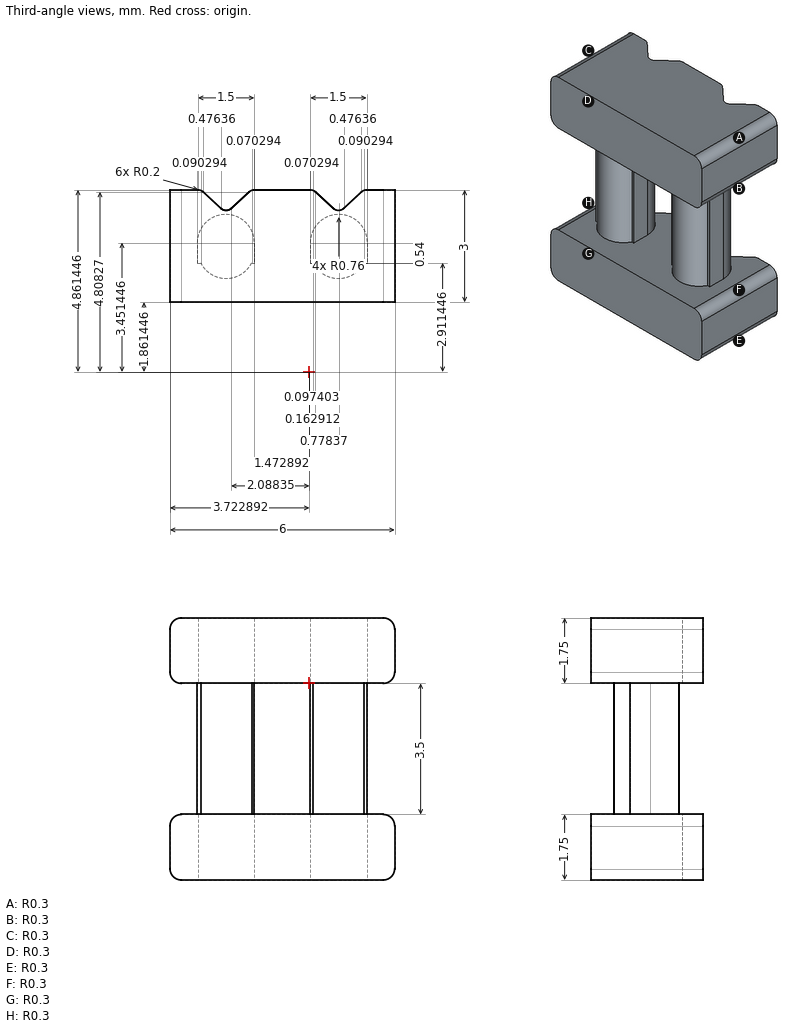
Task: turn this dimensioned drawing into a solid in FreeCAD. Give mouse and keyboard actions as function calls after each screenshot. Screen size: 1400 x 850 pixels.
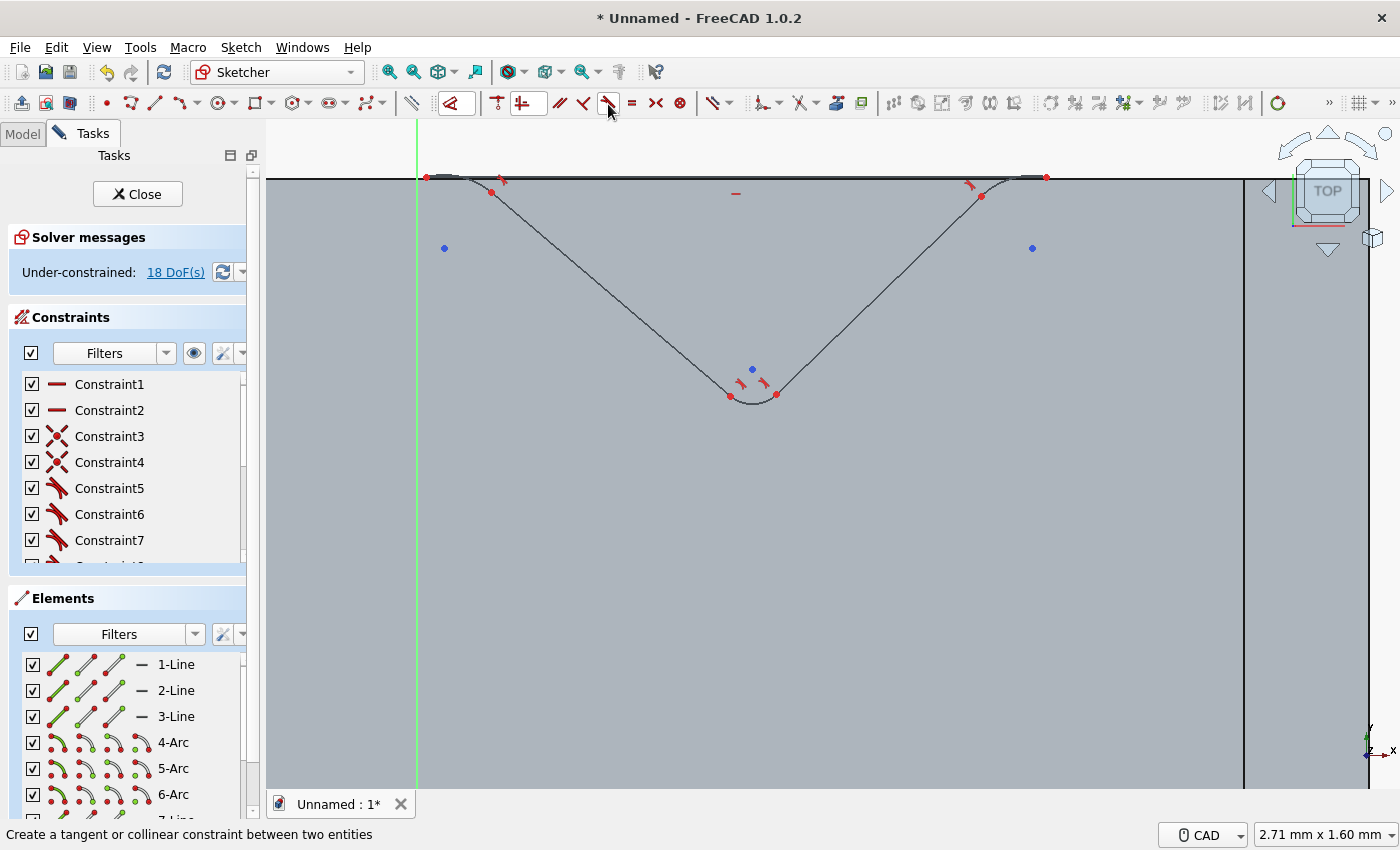
scroll(929, 267, down, 8)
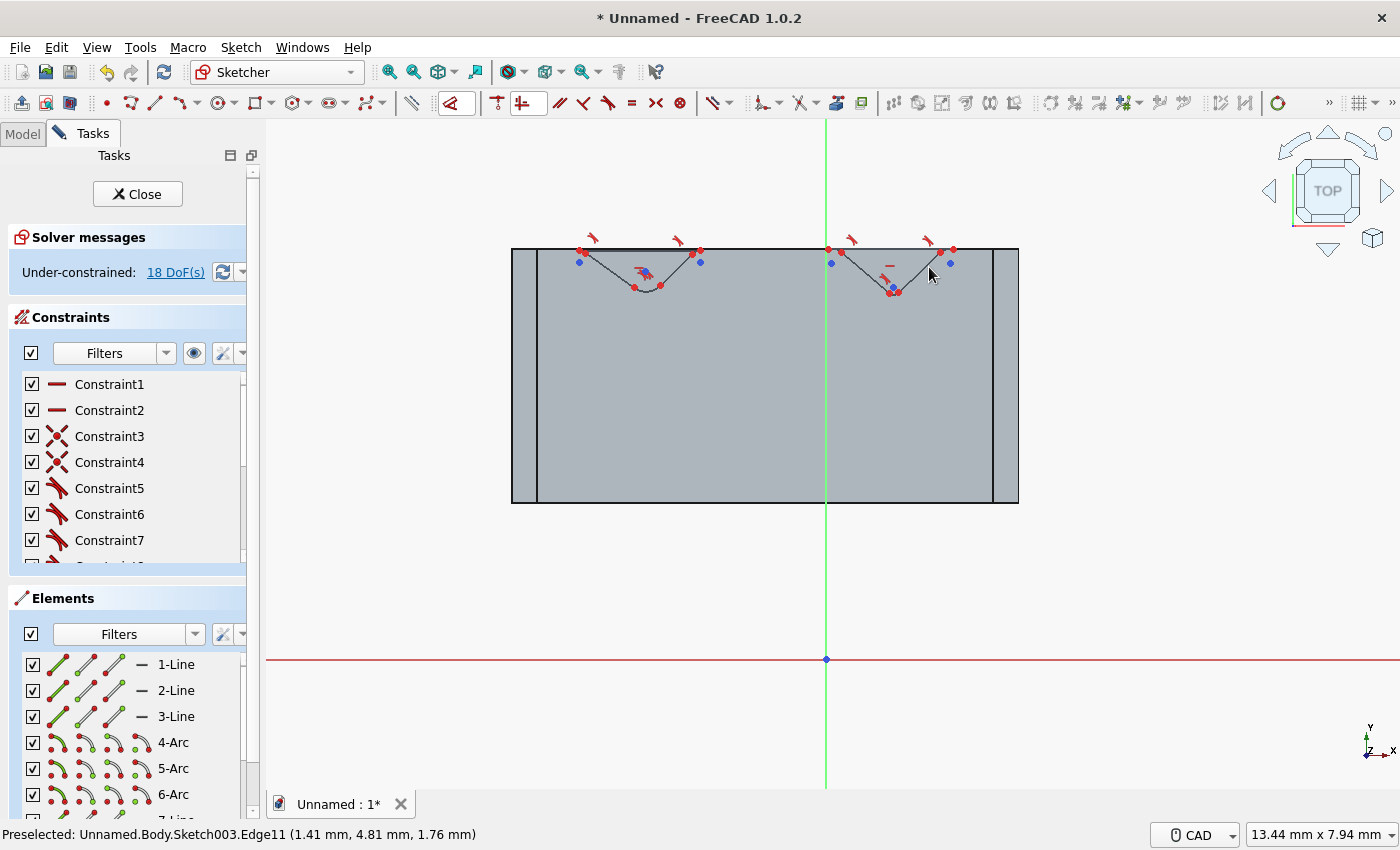
click(916, 249)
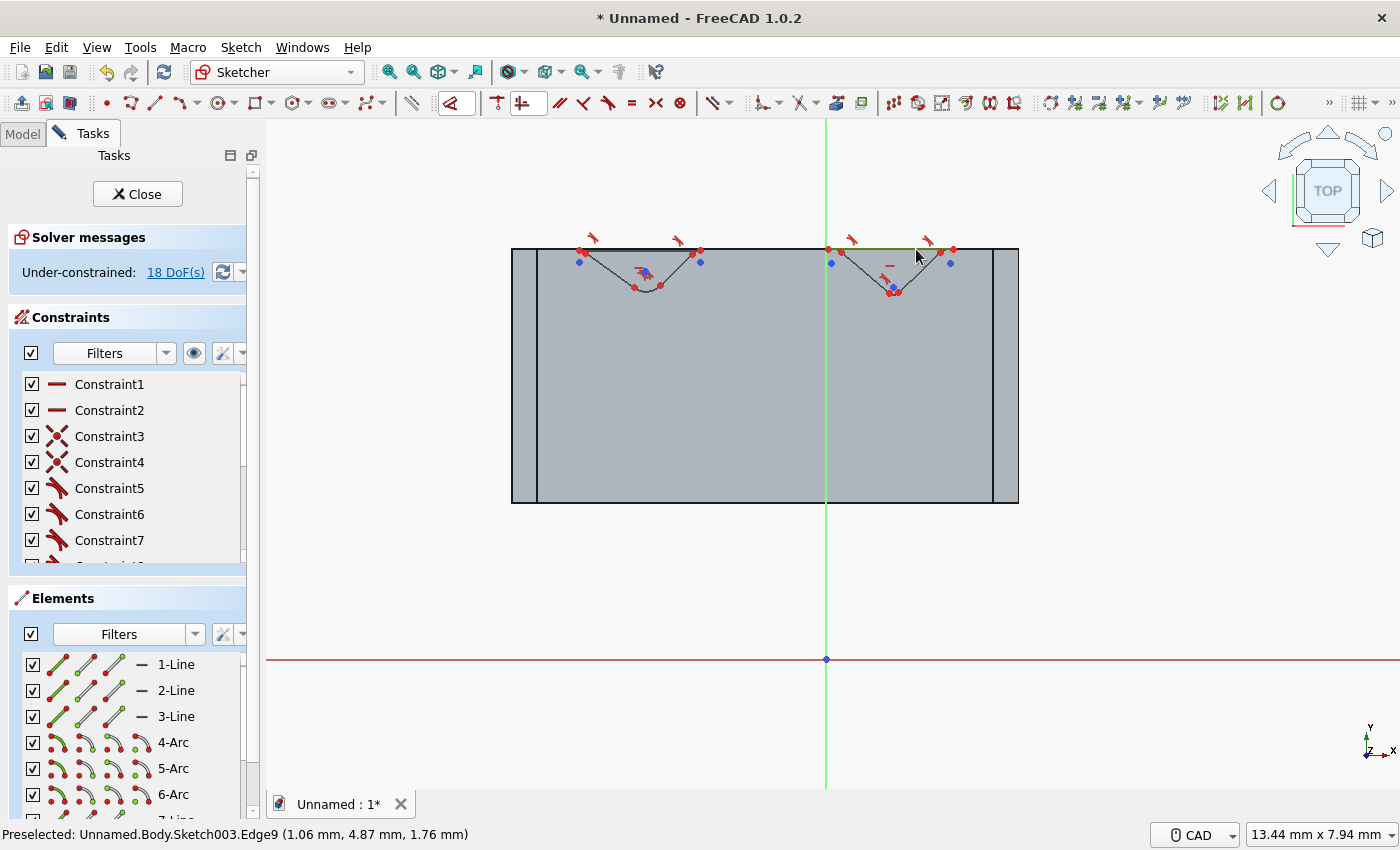
scroll(942, 251, up, 10)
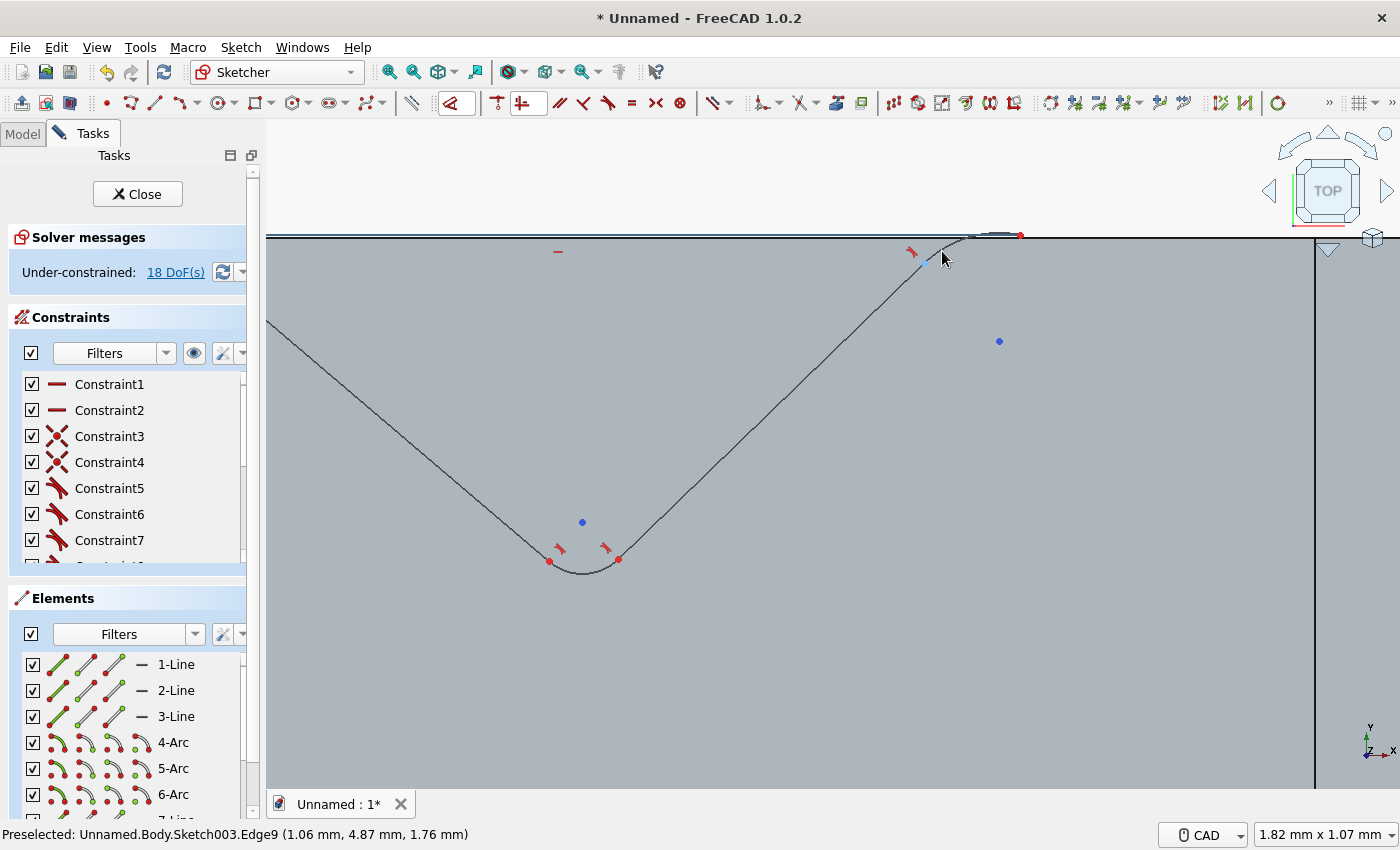
click(941, 250)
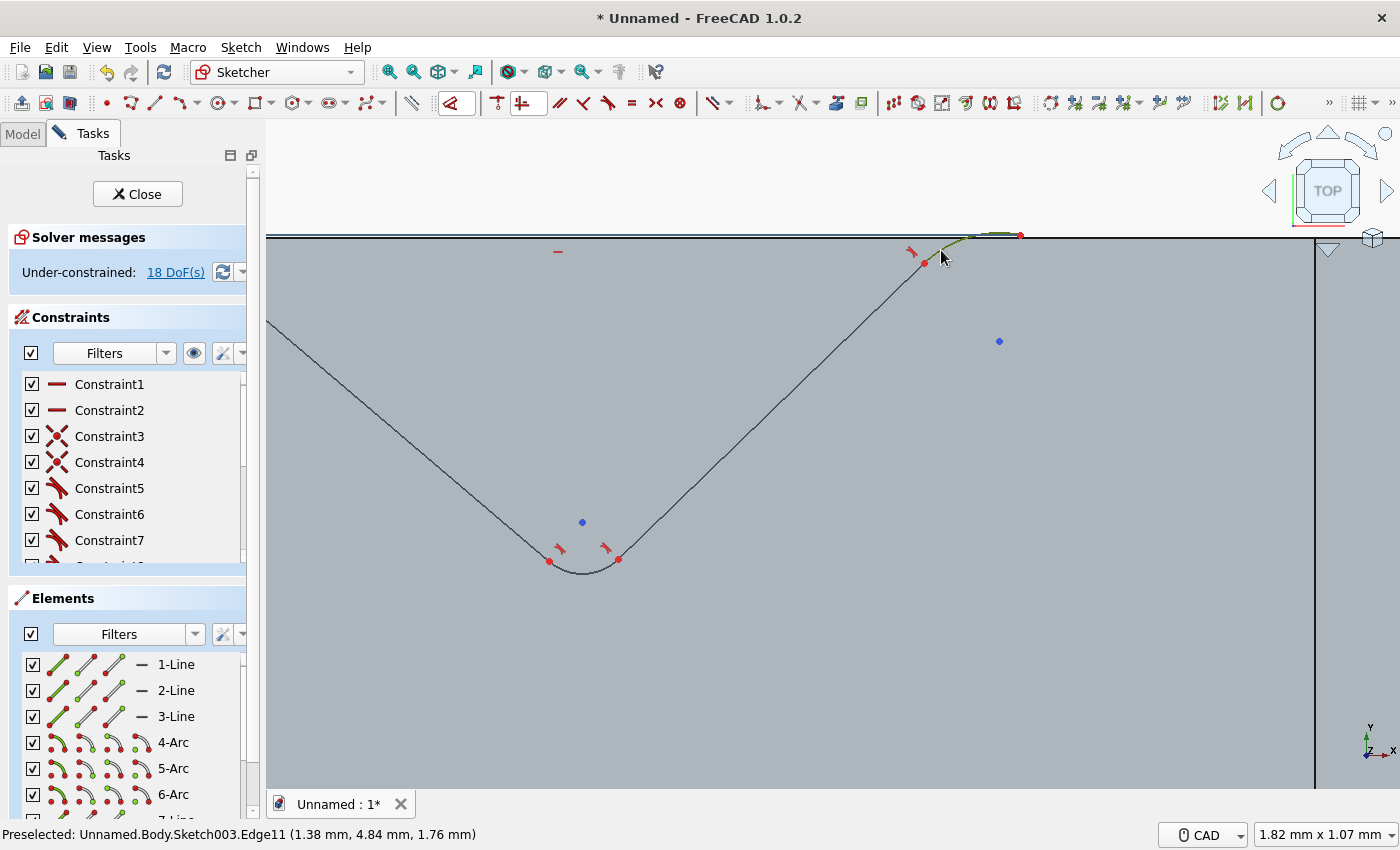
click(608, 104)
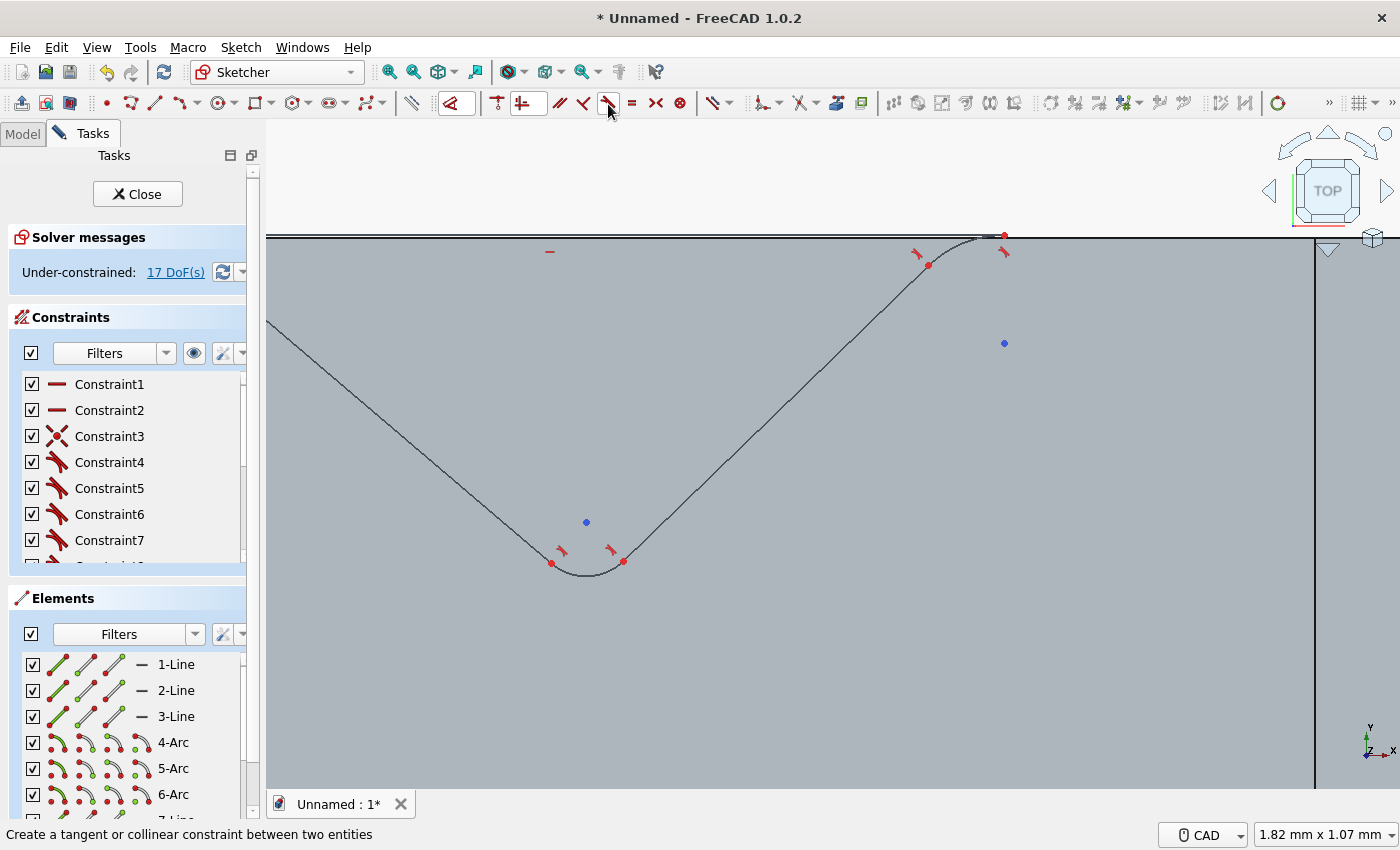
scroll(942, 251, down, 10)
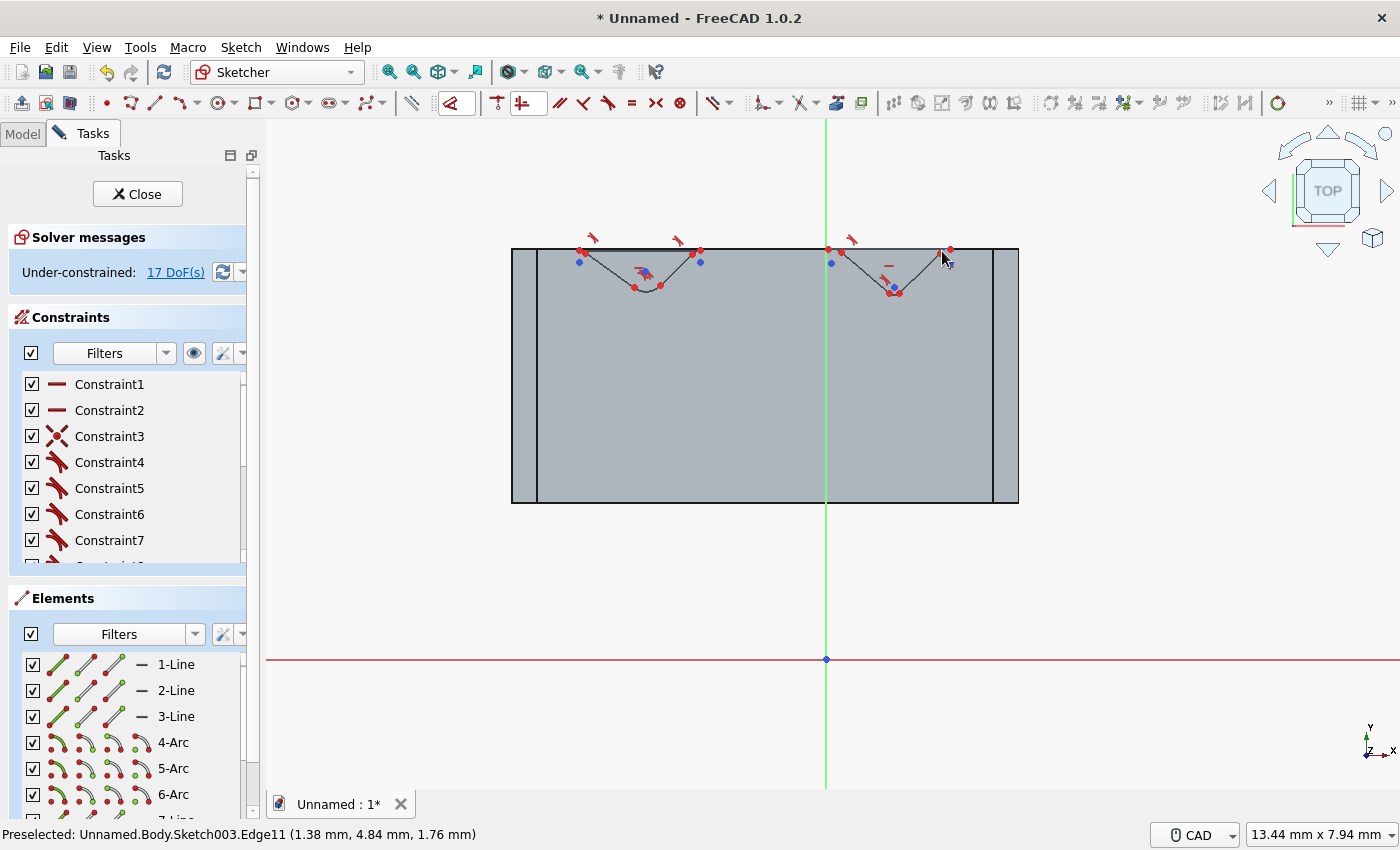
click(914, 249)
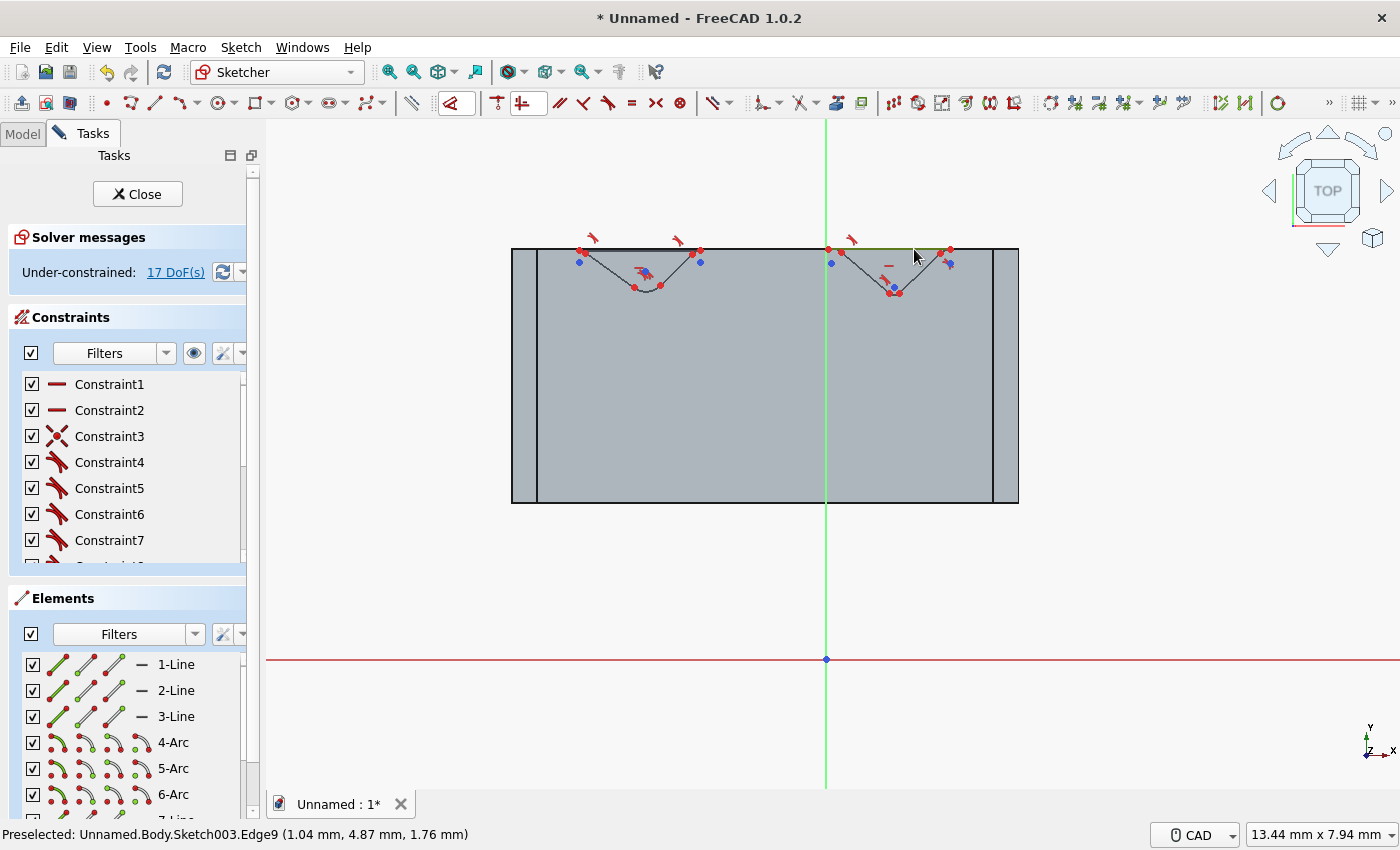
scroll(839, 251, up, 11)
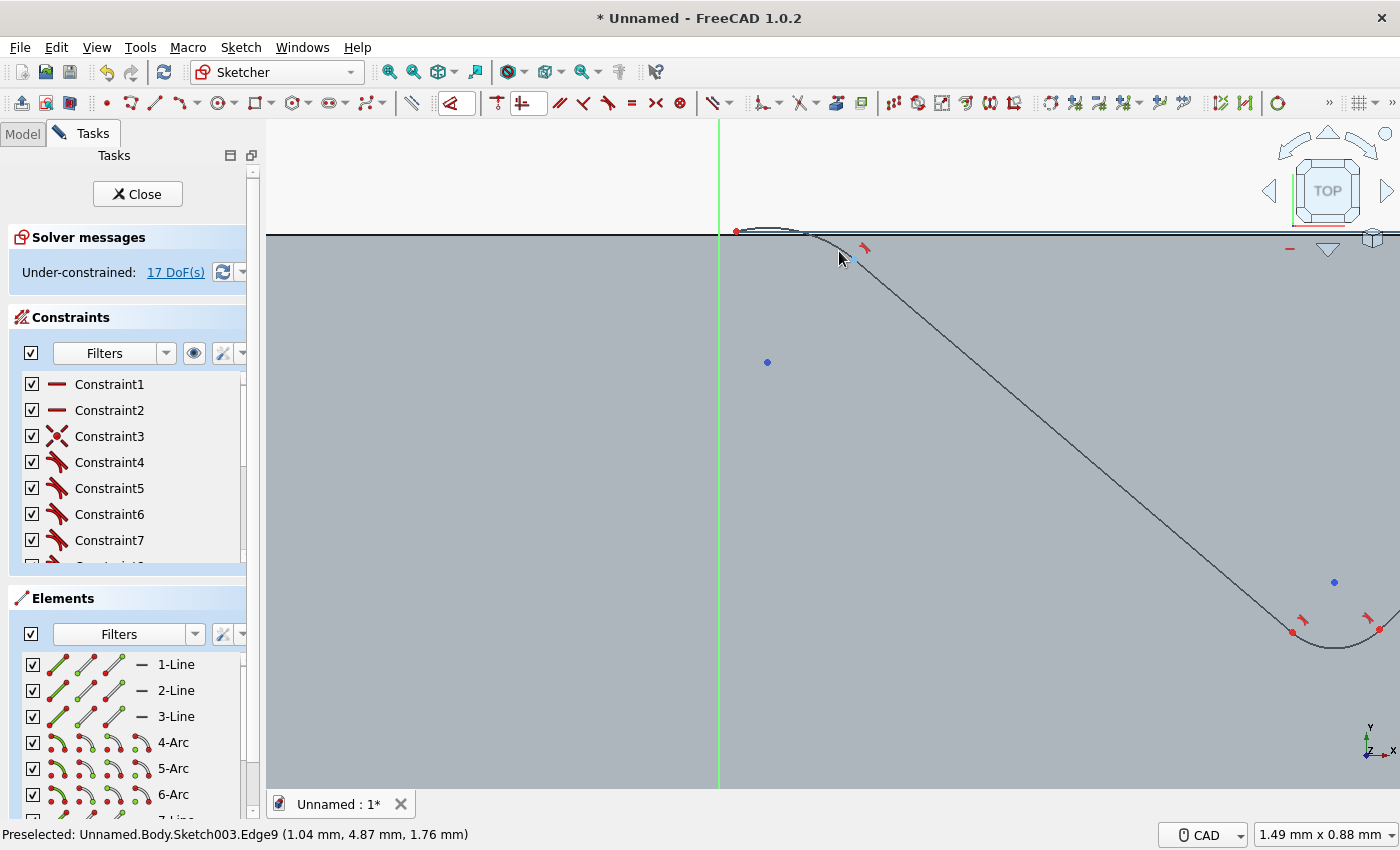
click(834, 245)